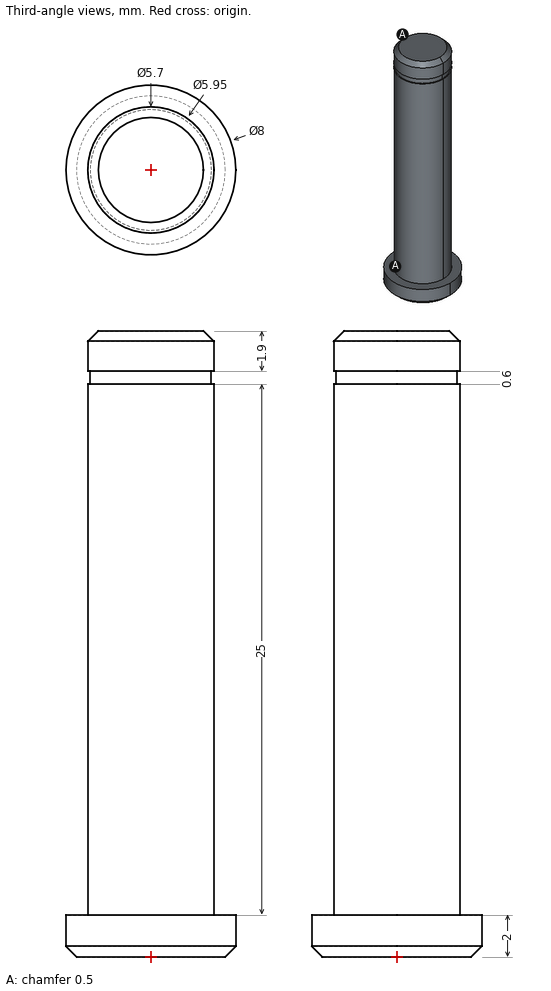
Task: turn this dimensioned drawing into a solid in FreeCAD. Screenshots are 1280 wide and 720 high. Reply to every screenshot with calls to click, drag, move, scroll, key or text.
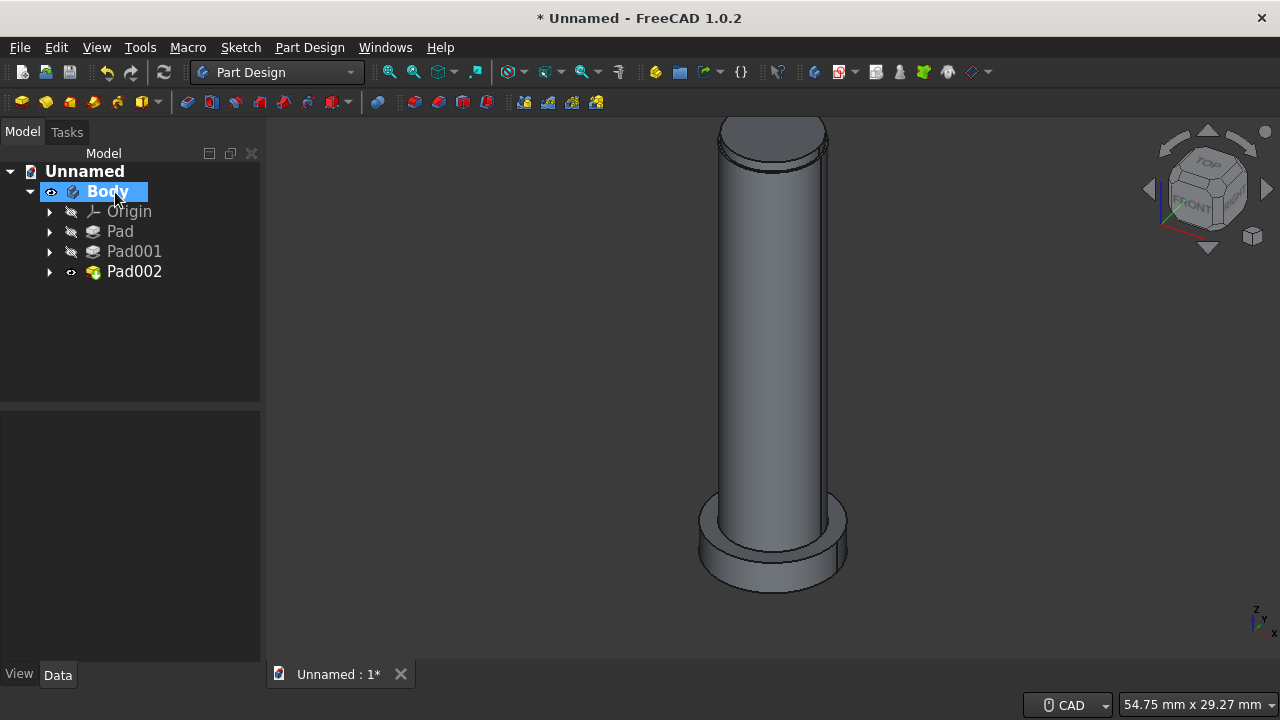
click(390, 72)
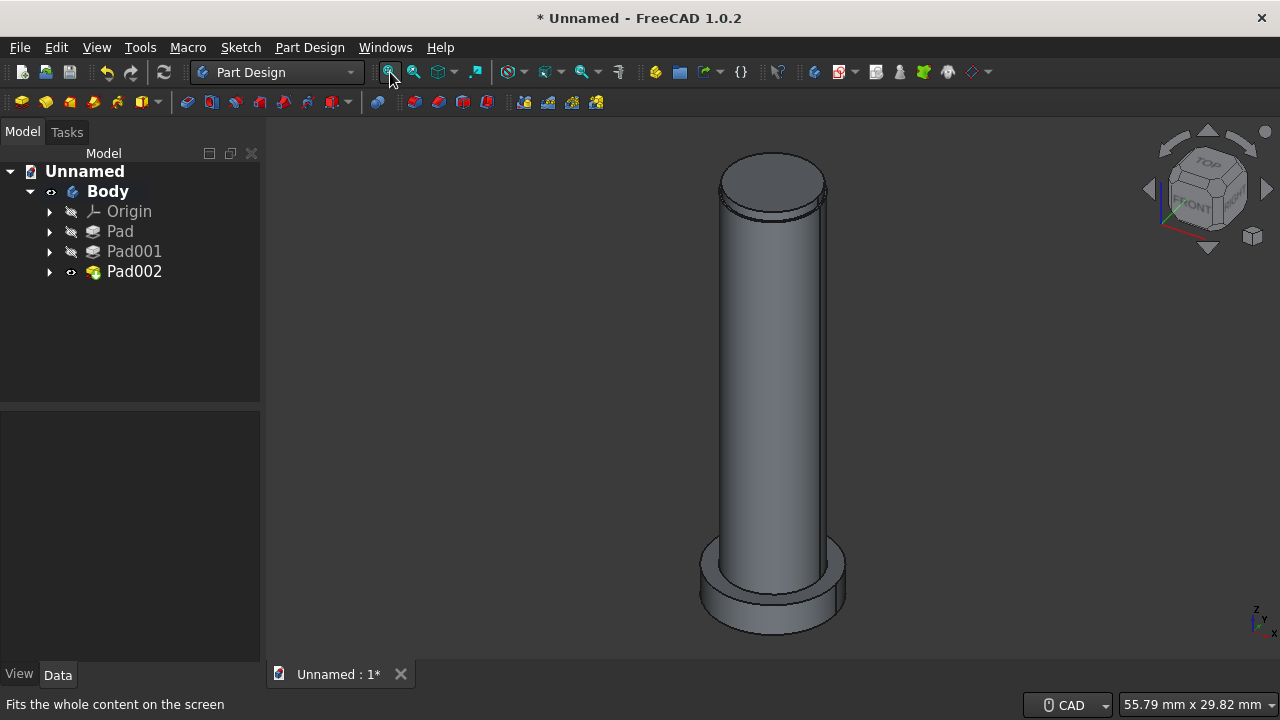
click(773, 182)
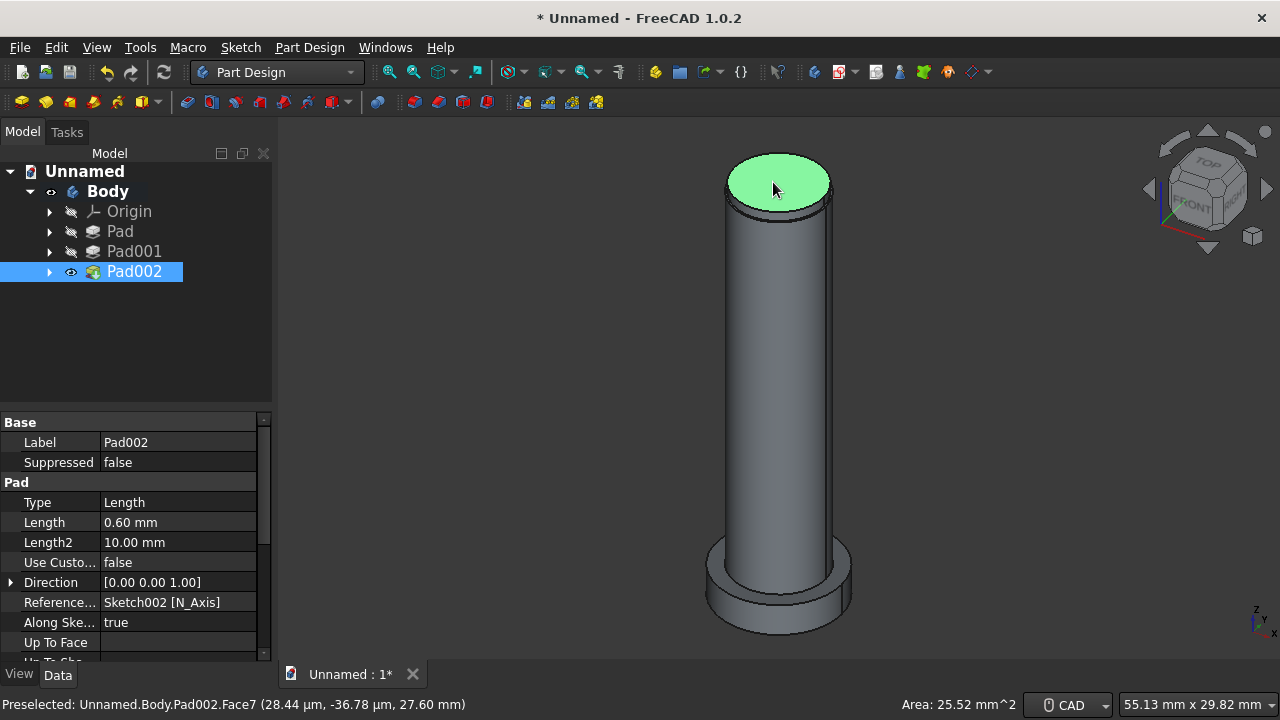
click(840, 72)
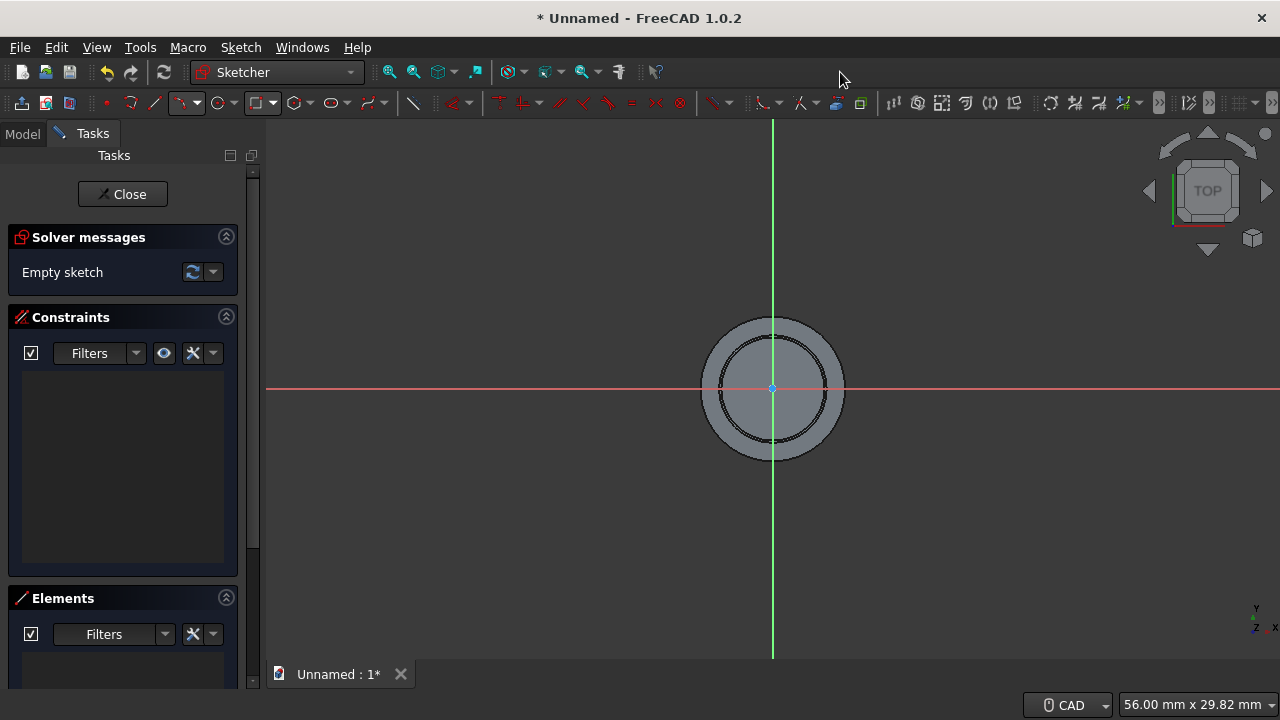
scroll(802, 389, up, 6)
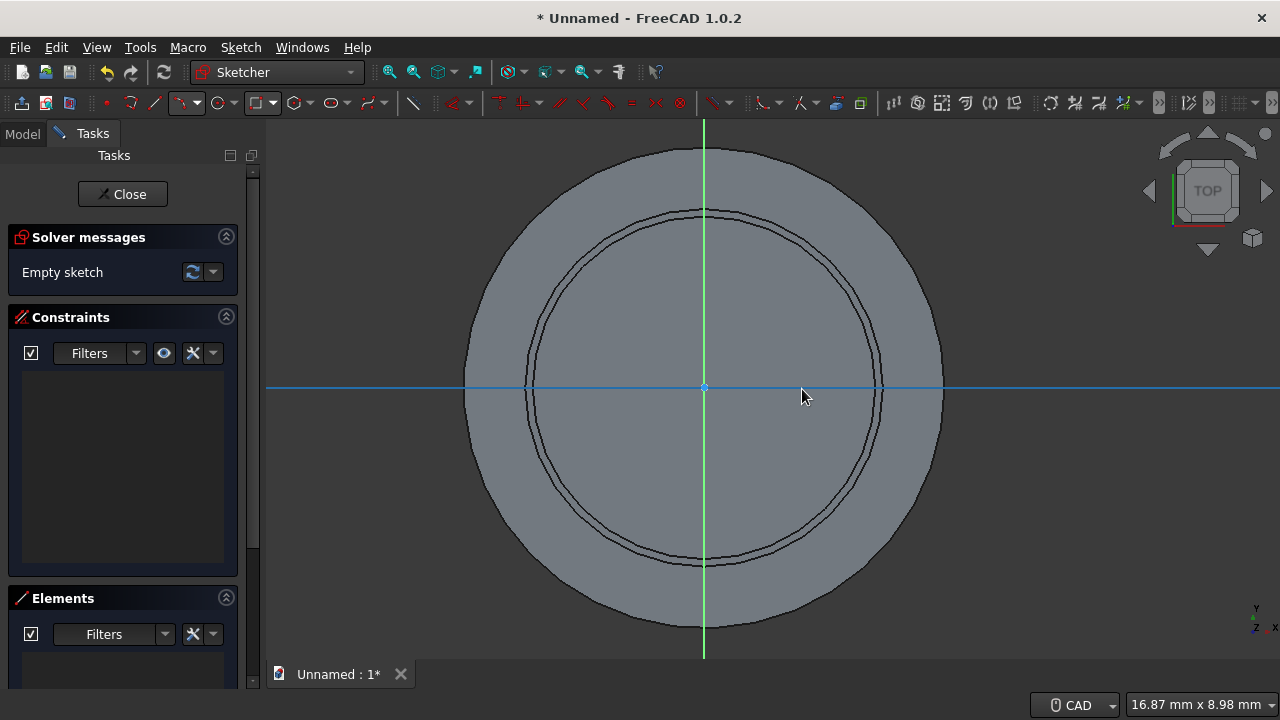
click(218, 104)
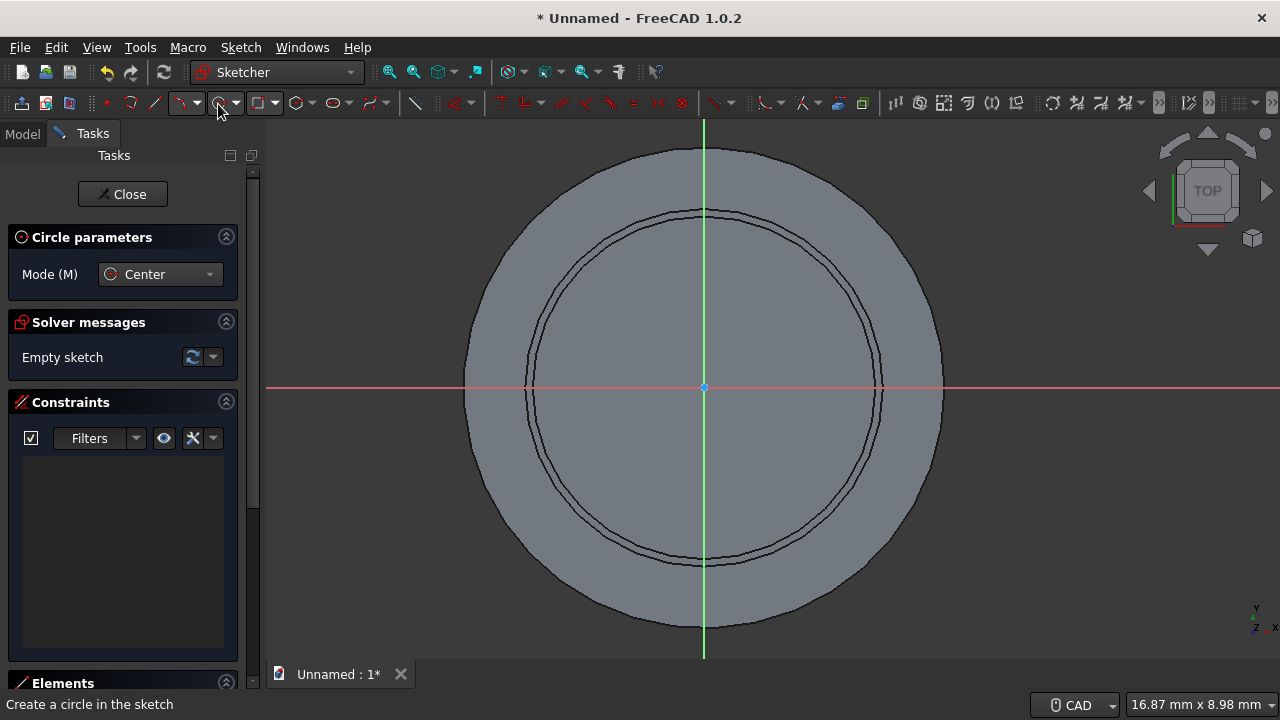
click(704, 388)
move(831, 261)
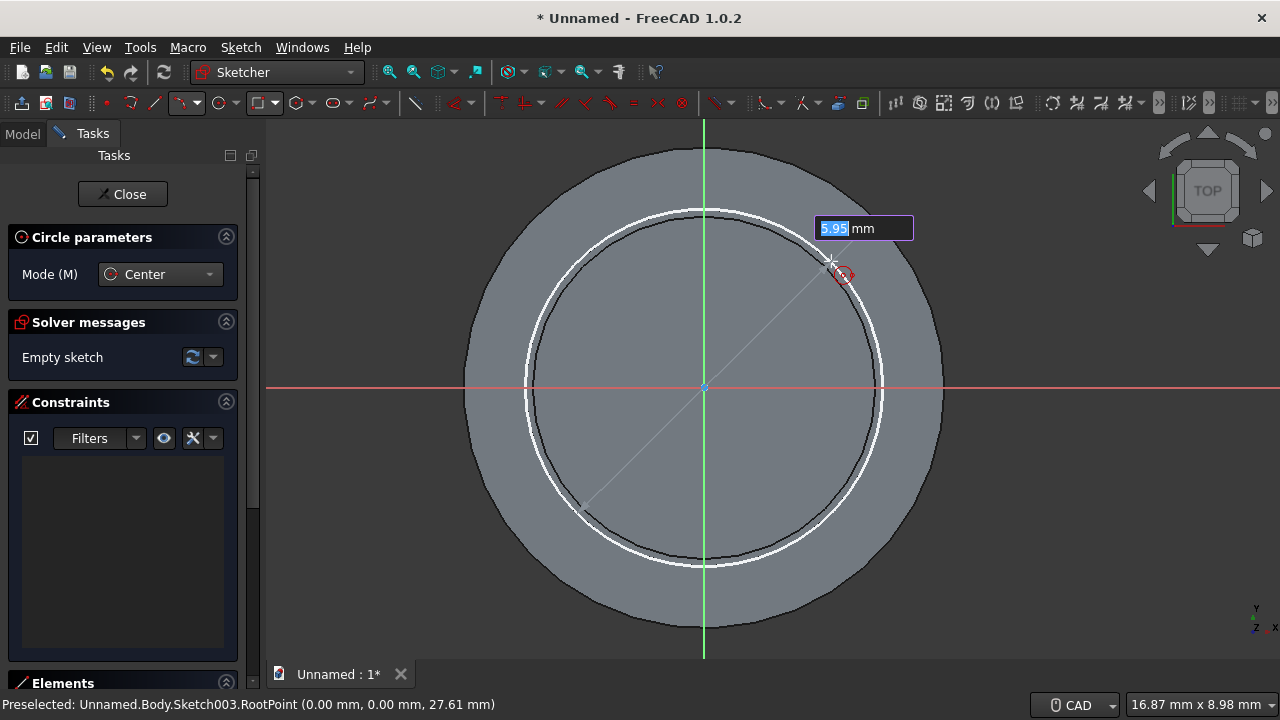
text(5.95)
key(Return)
key(Escape)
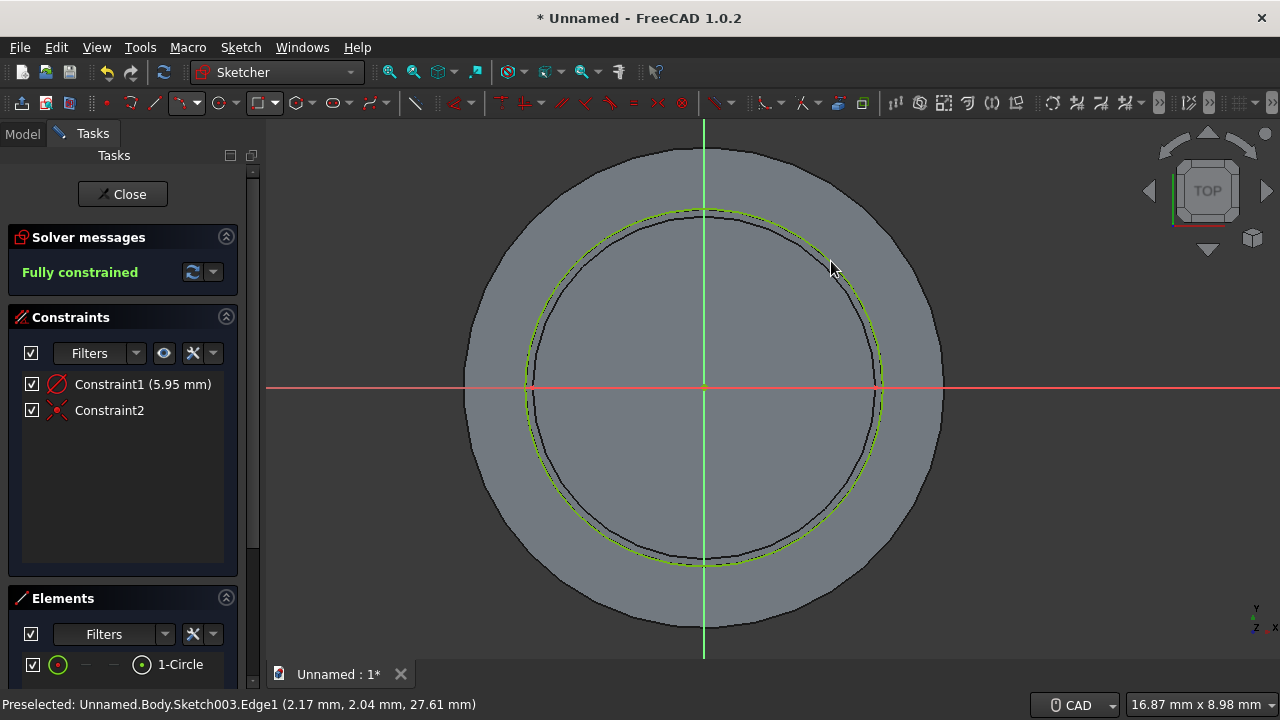
click(123, 194)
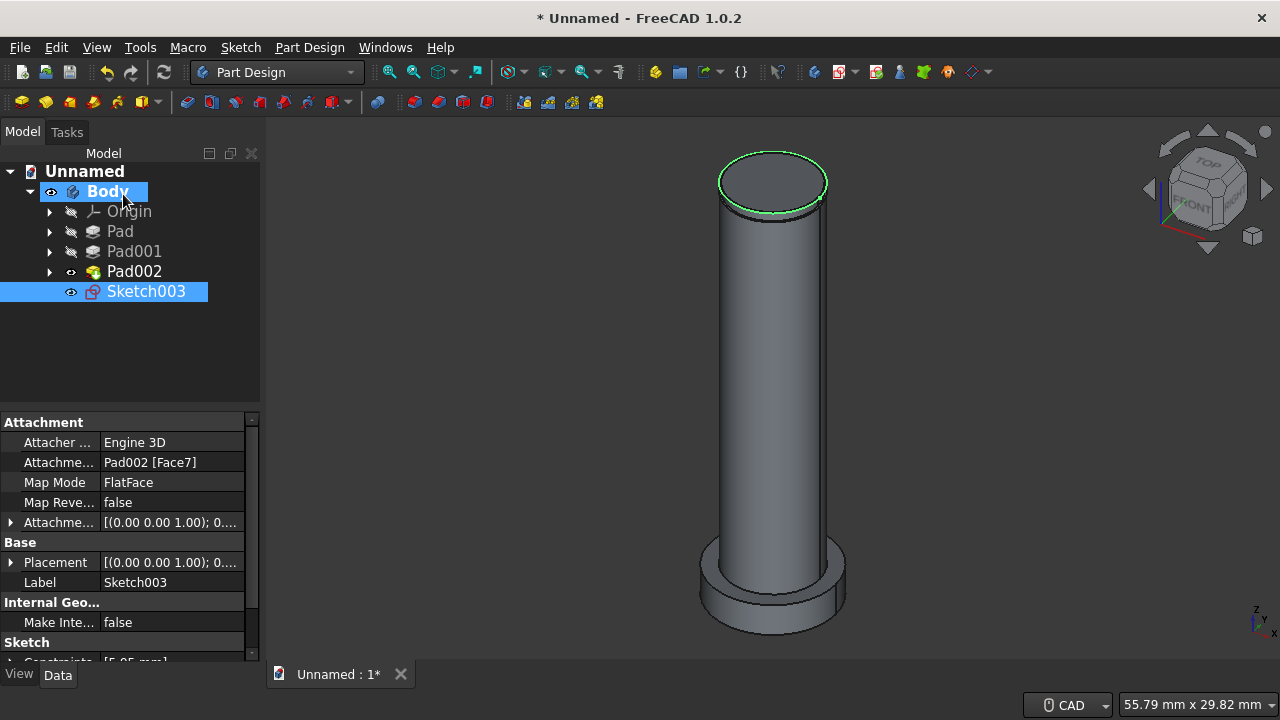
click(22, 102)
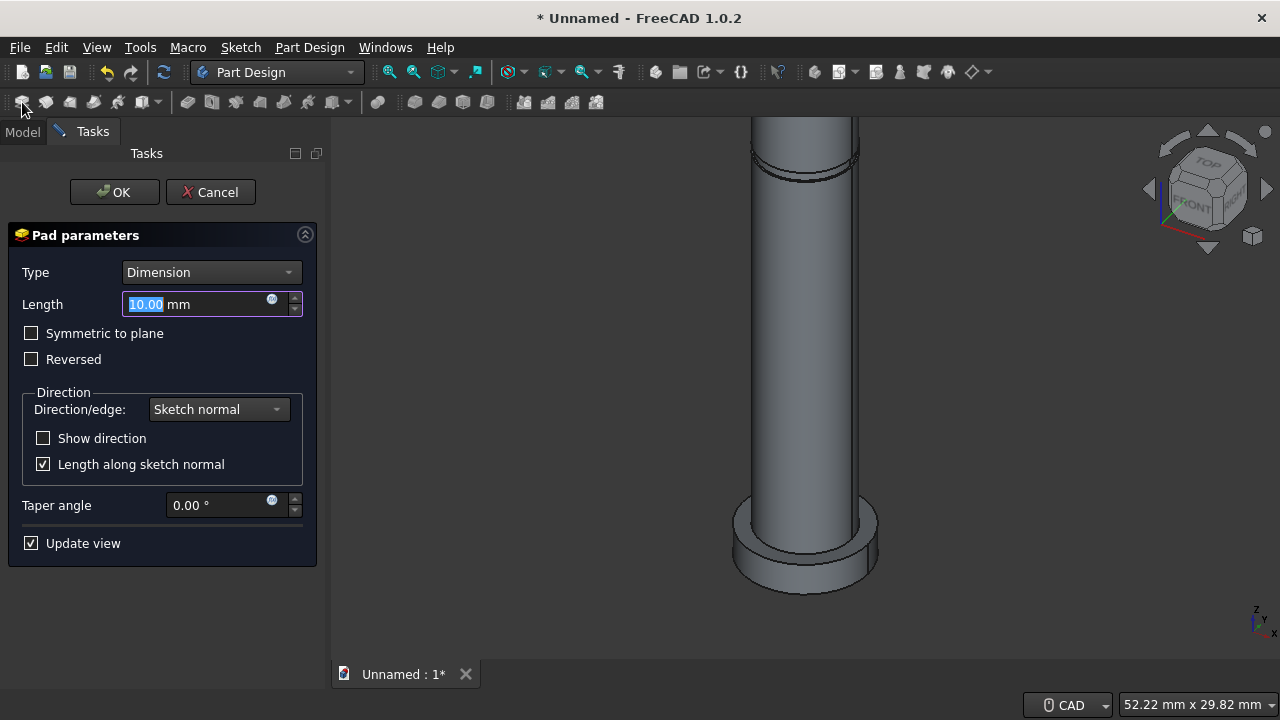
text(1.9)
key(Tab)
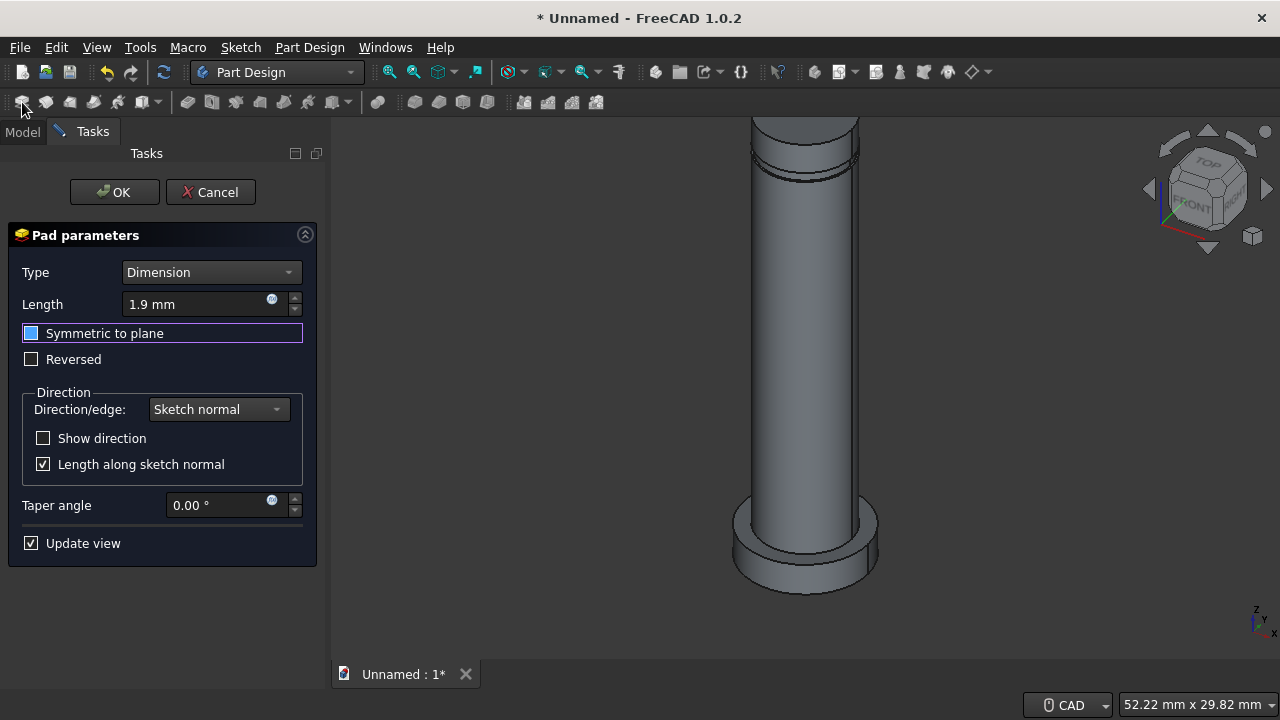
click(115, 192)